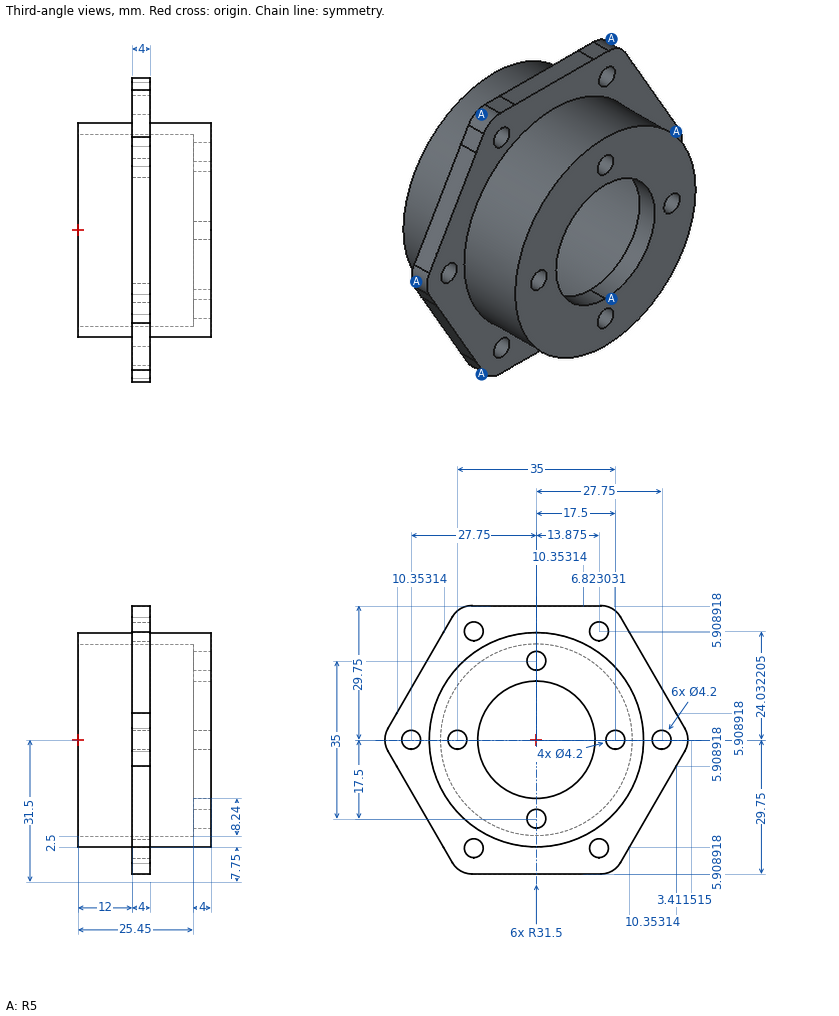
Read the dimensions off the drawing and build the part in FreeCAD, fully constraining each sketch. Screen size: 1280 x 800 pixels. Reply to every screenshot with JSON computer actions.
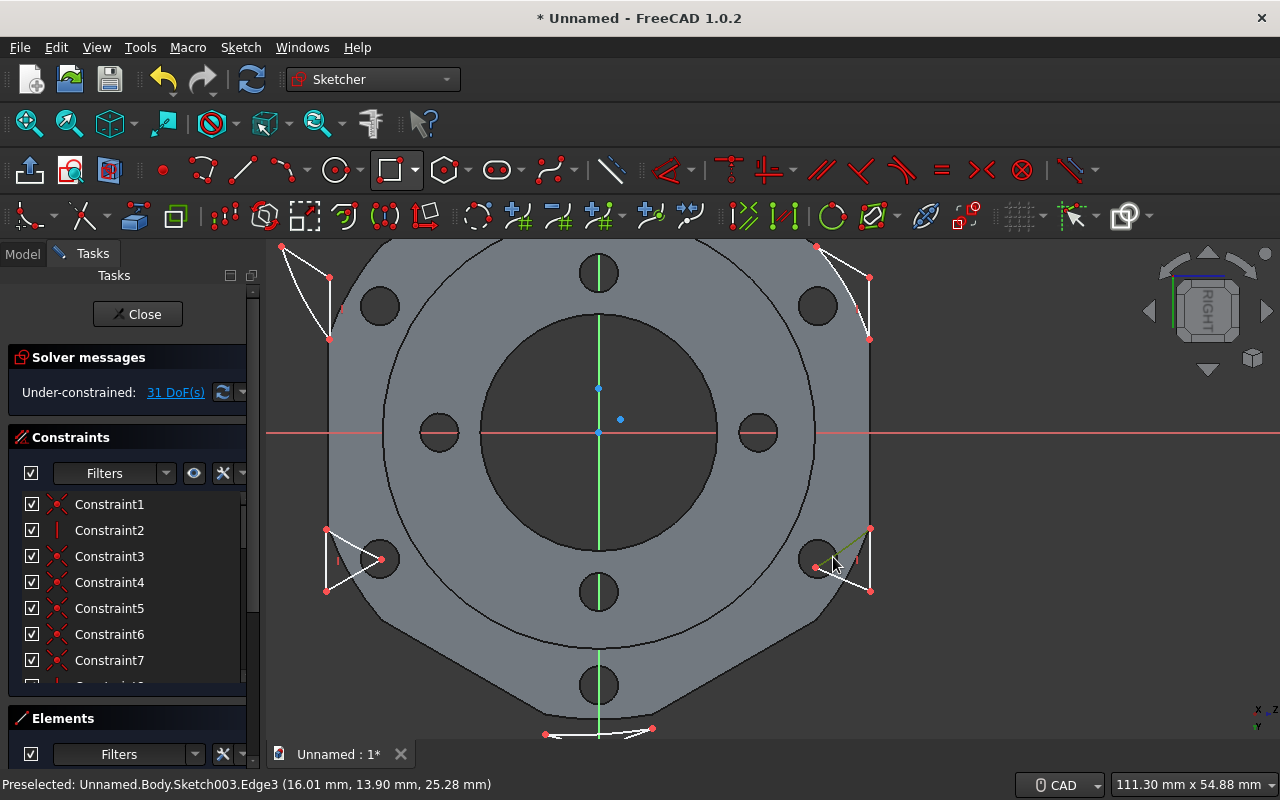
{"action": "scroll", "coordinate": [833, 558], "scroll_direction": "down", "scroll_amount": 3}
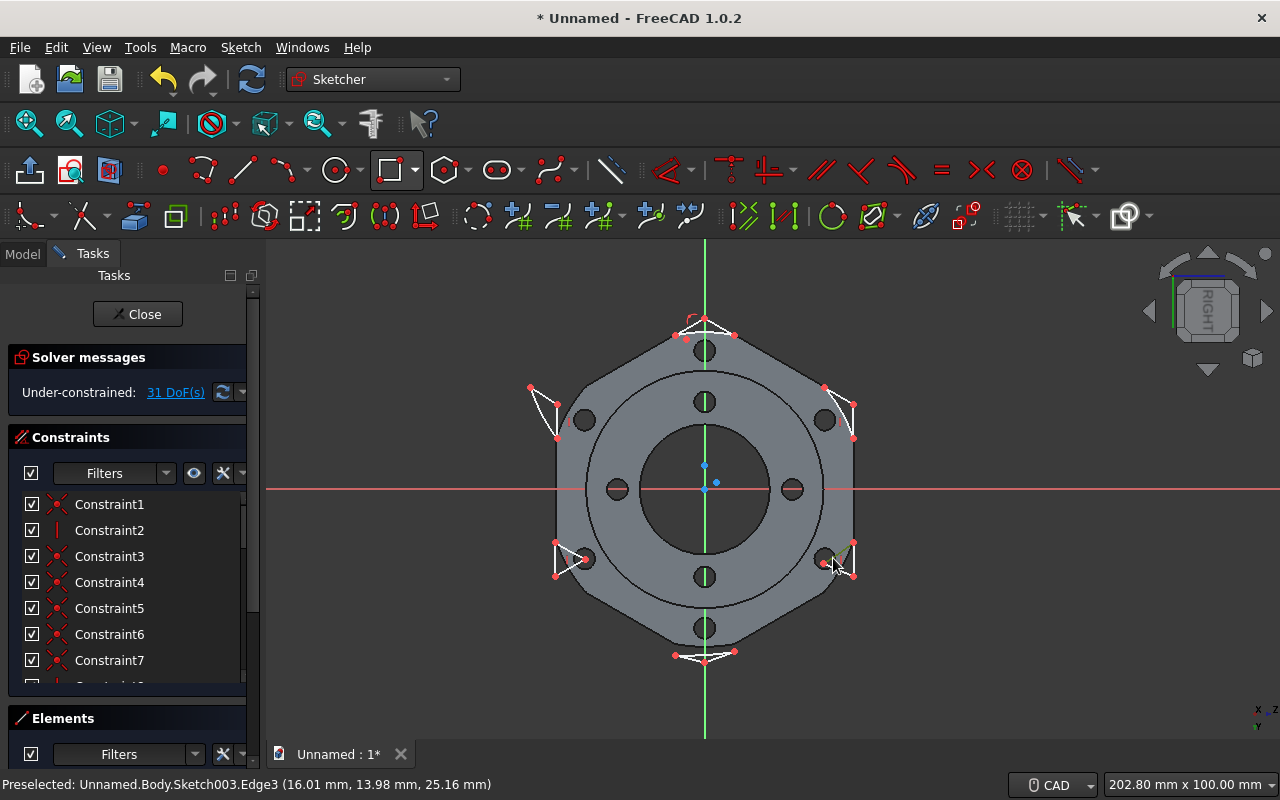
{"action": "scroll", "coordinate": [717, 333], "scroll_direction": "up", "scroll_amount": 4}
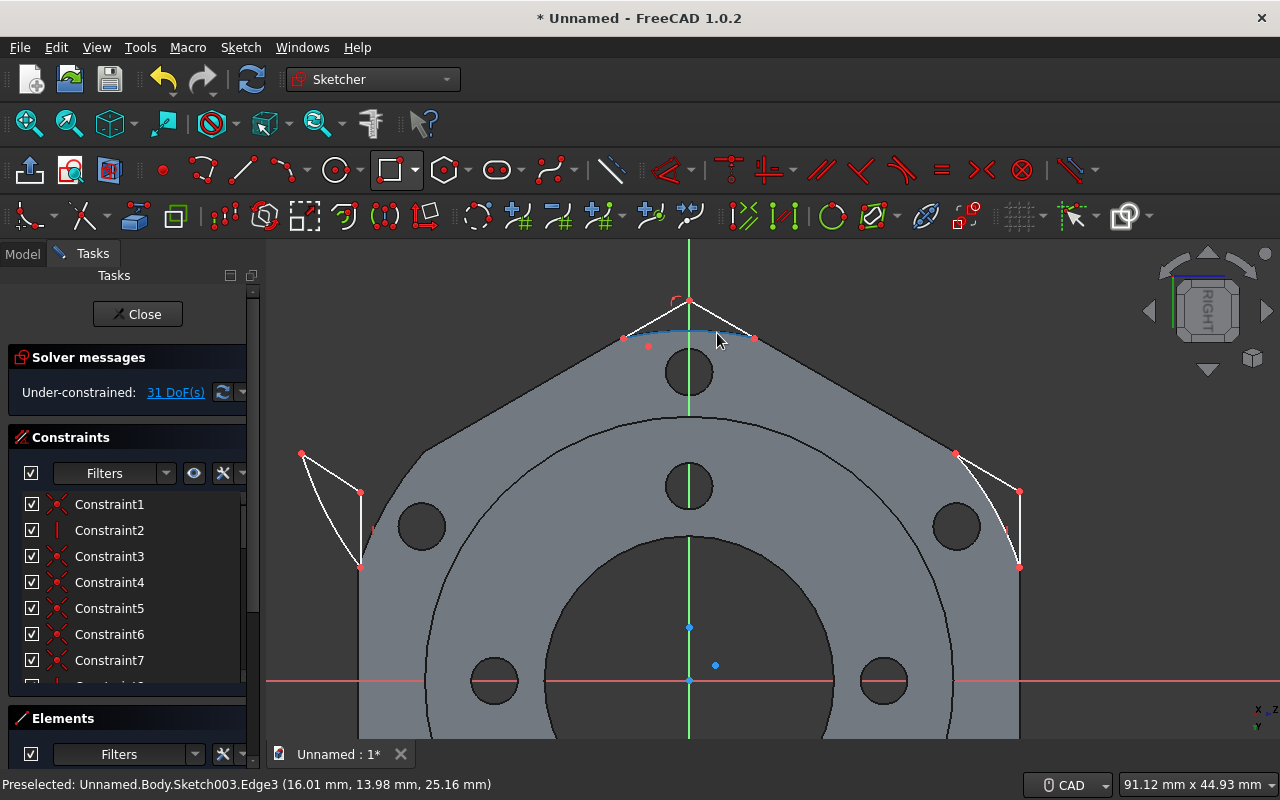
{"action": "left_click", "coordinate": [716, 332]}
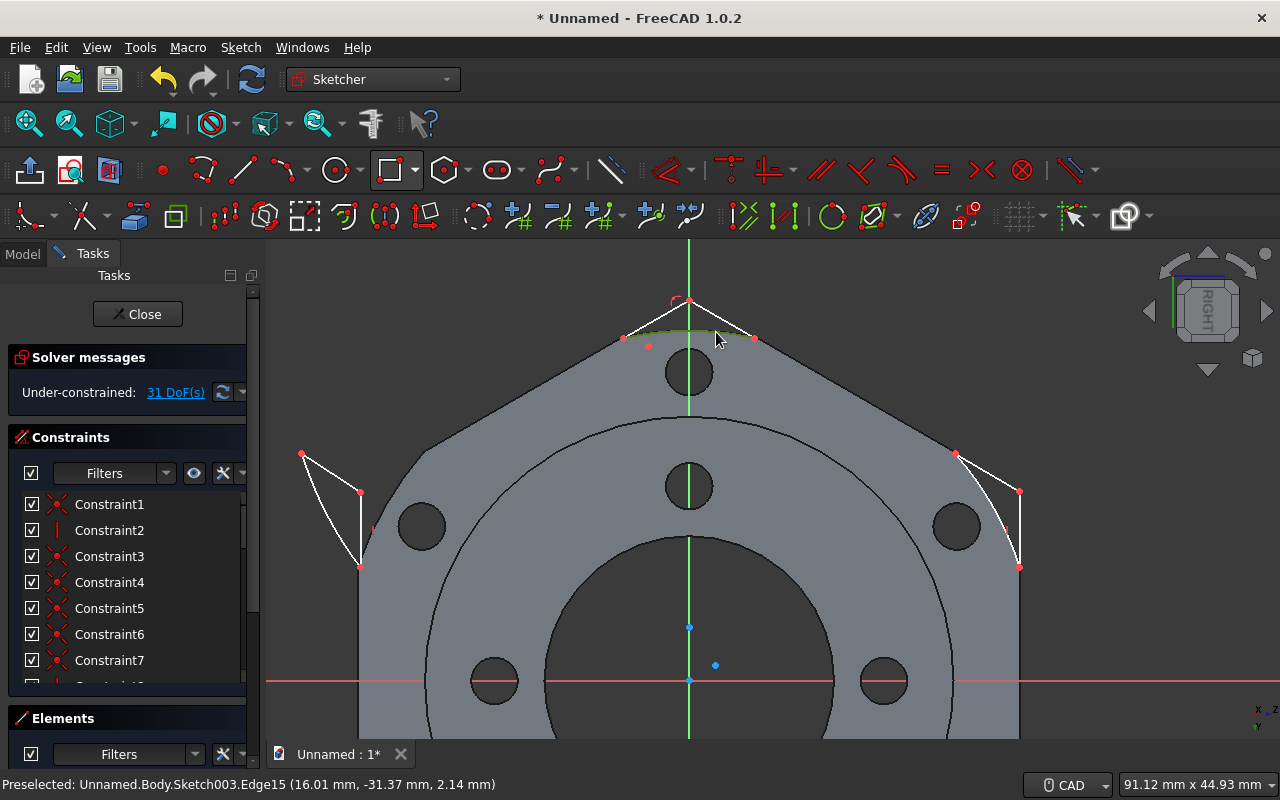
{"action": "key", "text": "c"}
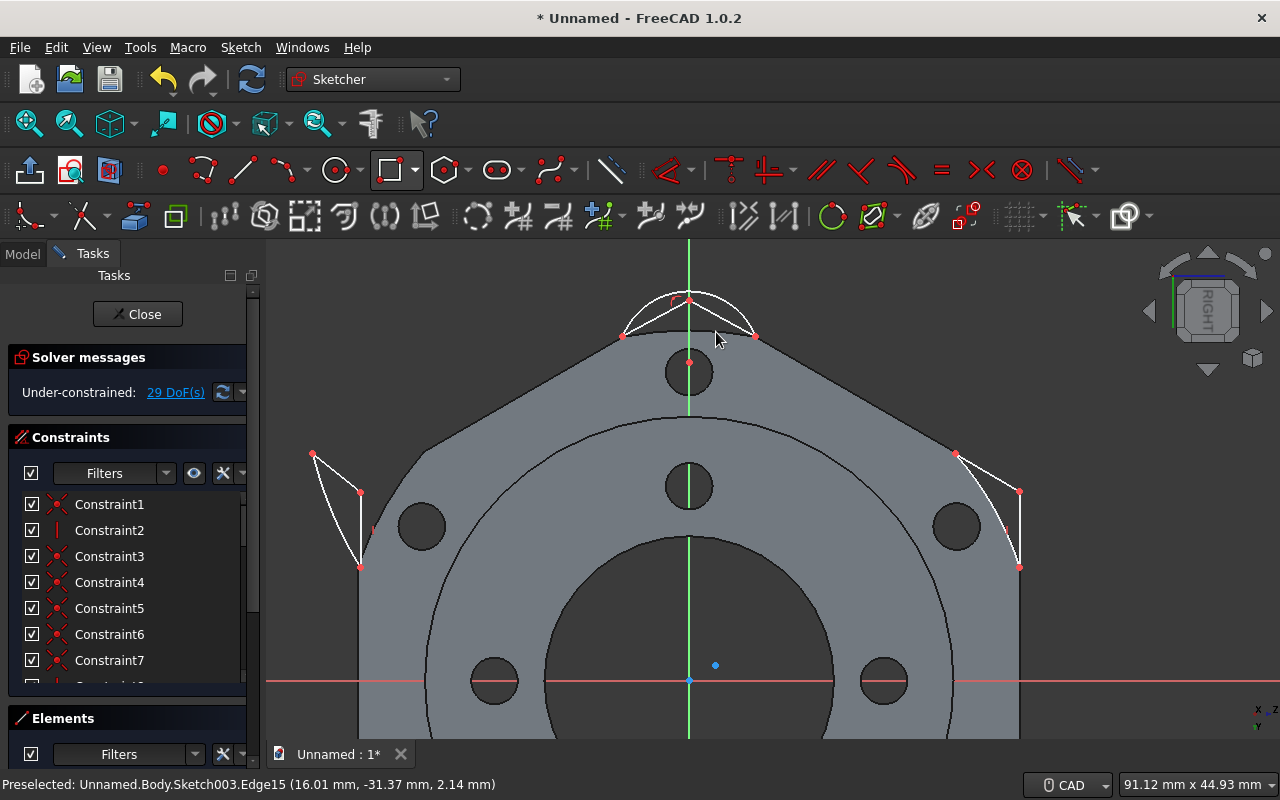
{"action": "scroll", "coordinate": [717, 332], "scroll_direction": "down", "scroll_amount": 4}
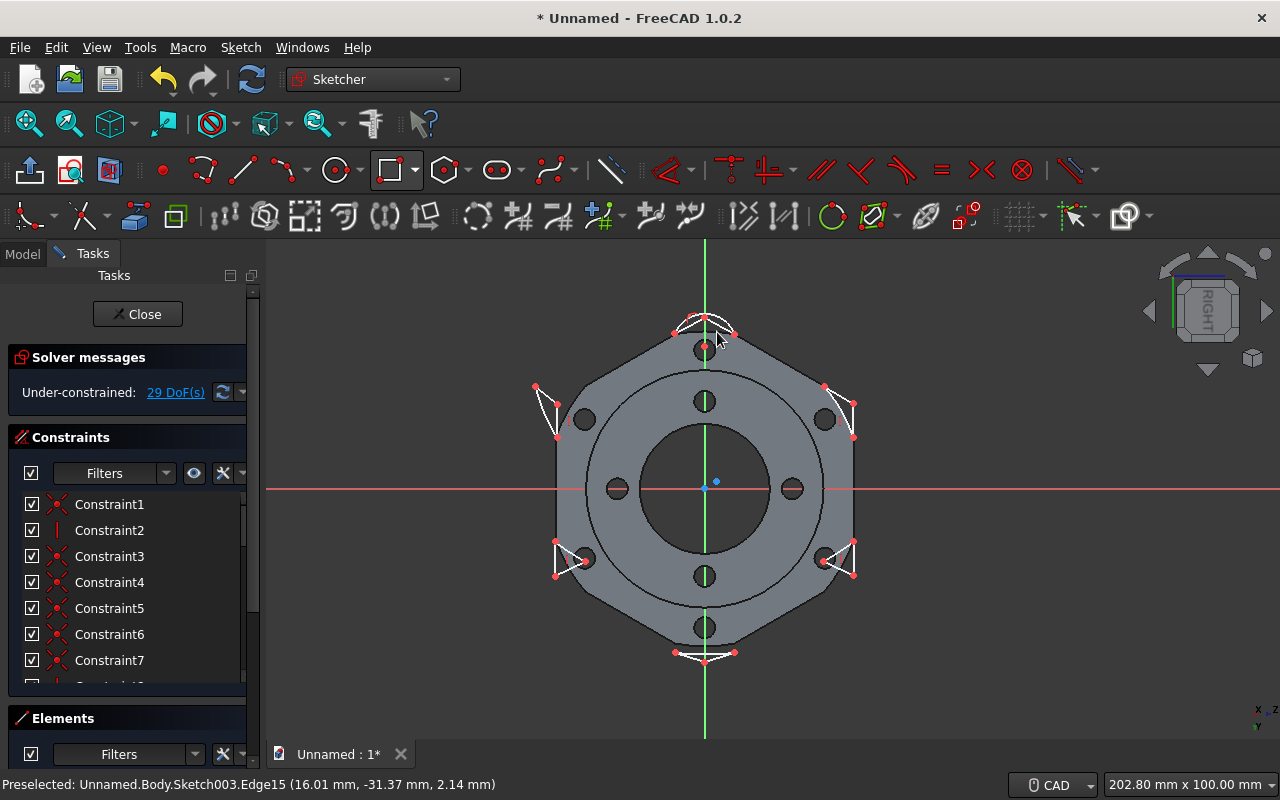
{"action": "scroll", "coordinate": [833, 556], "scroll_direction": "up", "scroll_amount": 3}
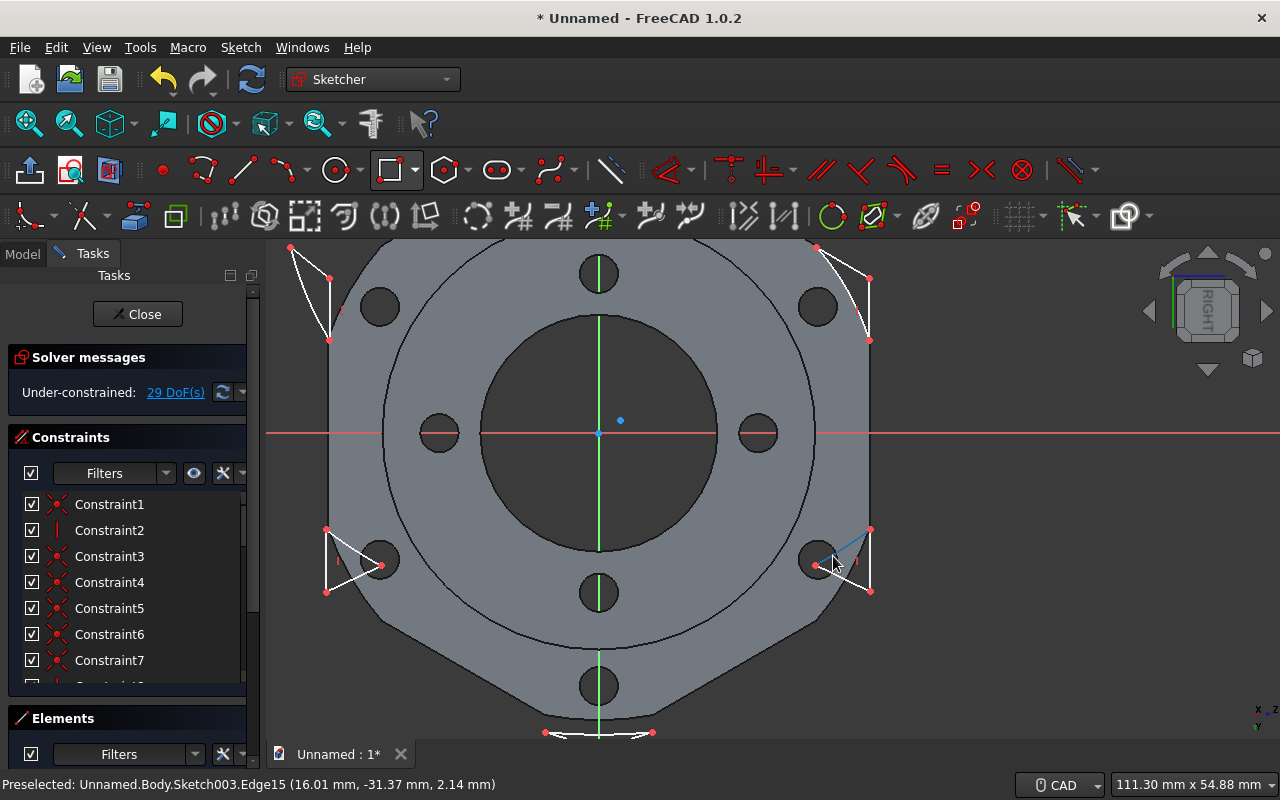
{"action": "left_click", "coordinate": [833, 555]}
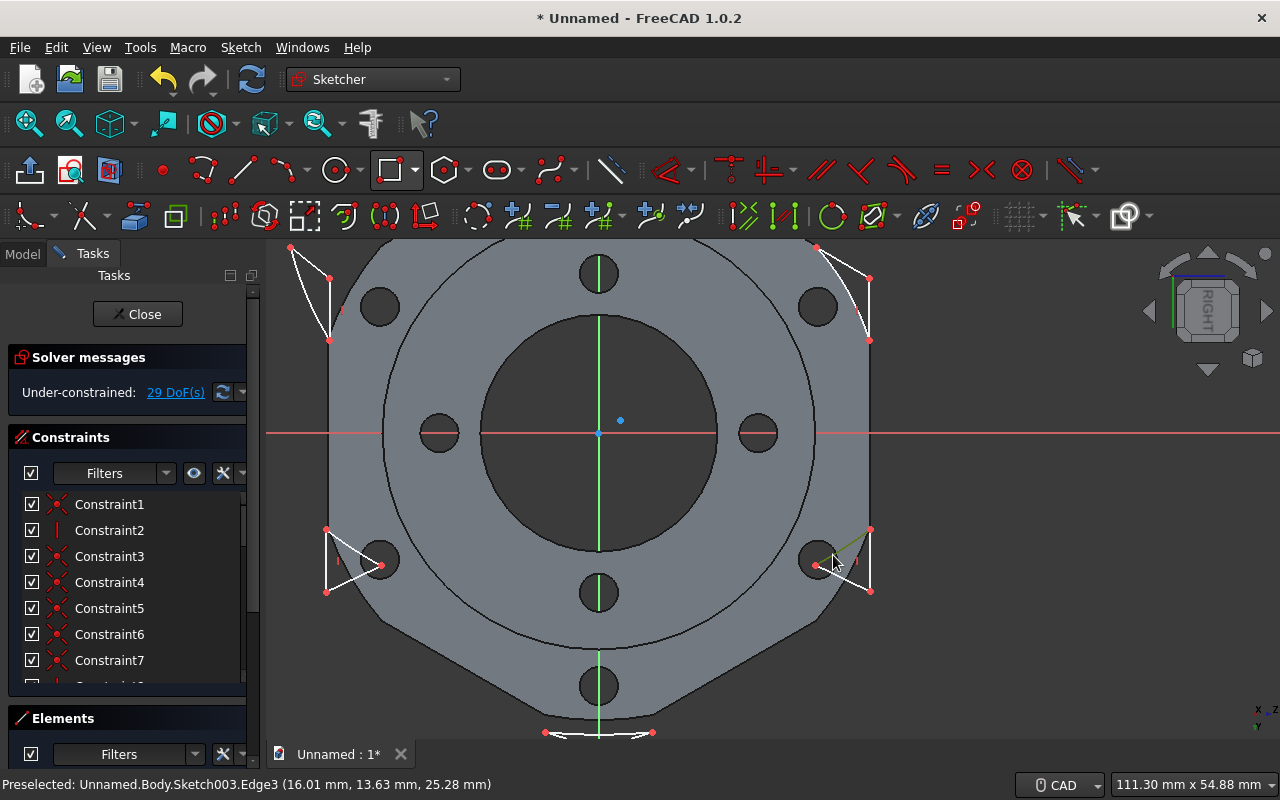
{"action": "left_click", "coordinate": [836, 273]}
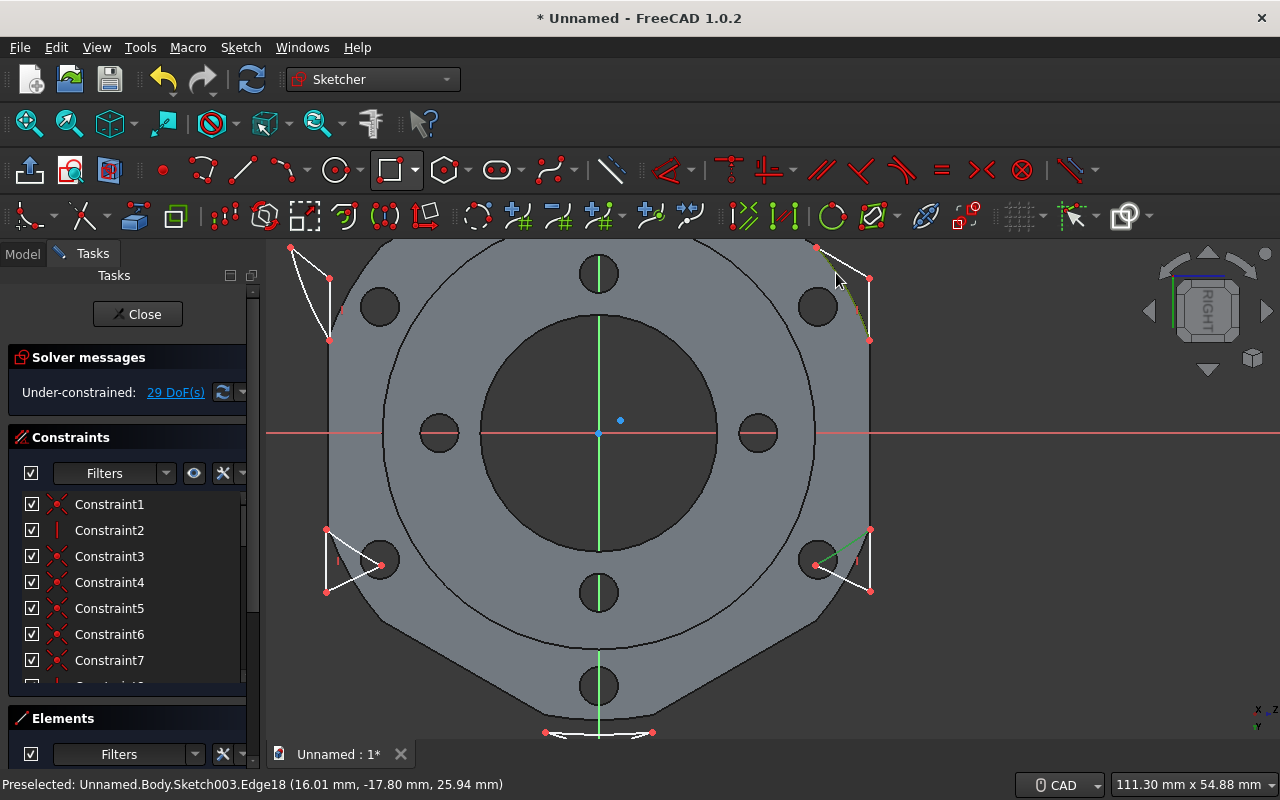
{"action": "key", "text": "c"}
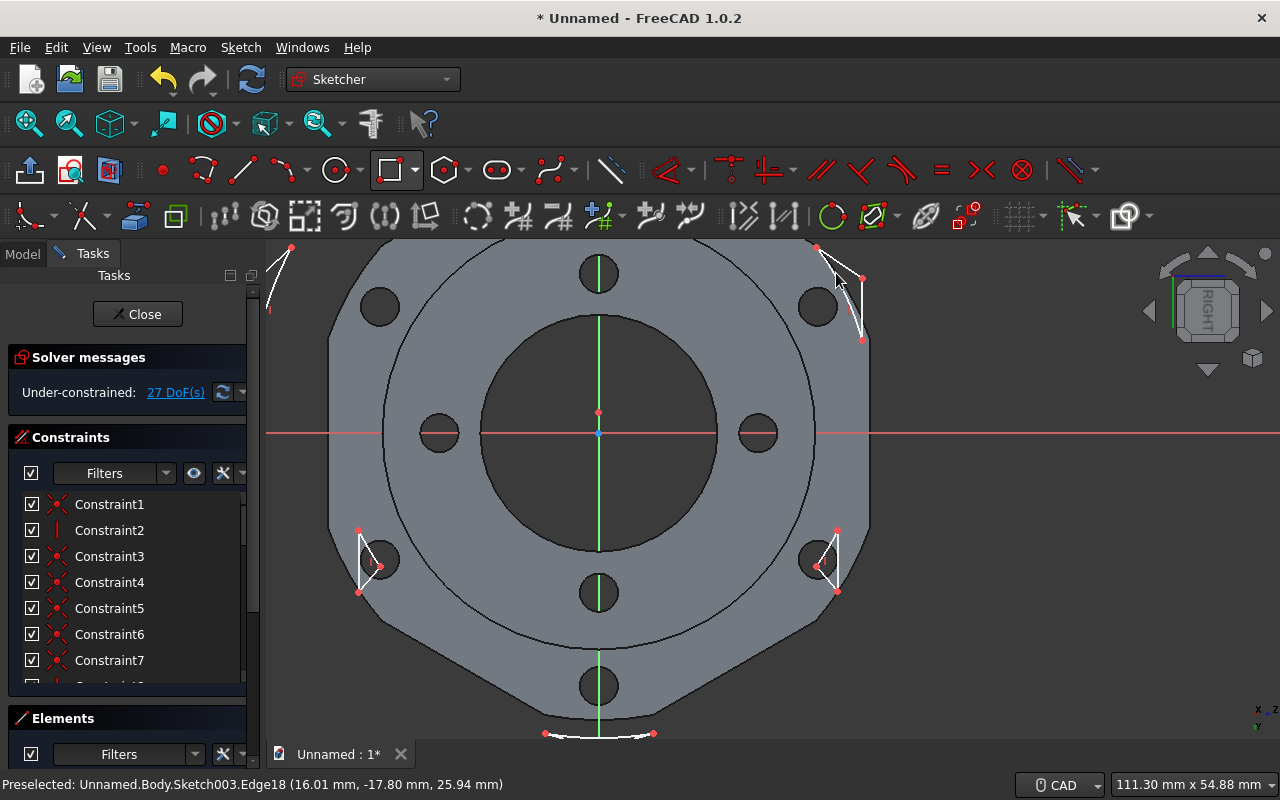
{"action": "left_click_drag", "start_coordinate": [589, 402], "coordinate": [609, 443]}